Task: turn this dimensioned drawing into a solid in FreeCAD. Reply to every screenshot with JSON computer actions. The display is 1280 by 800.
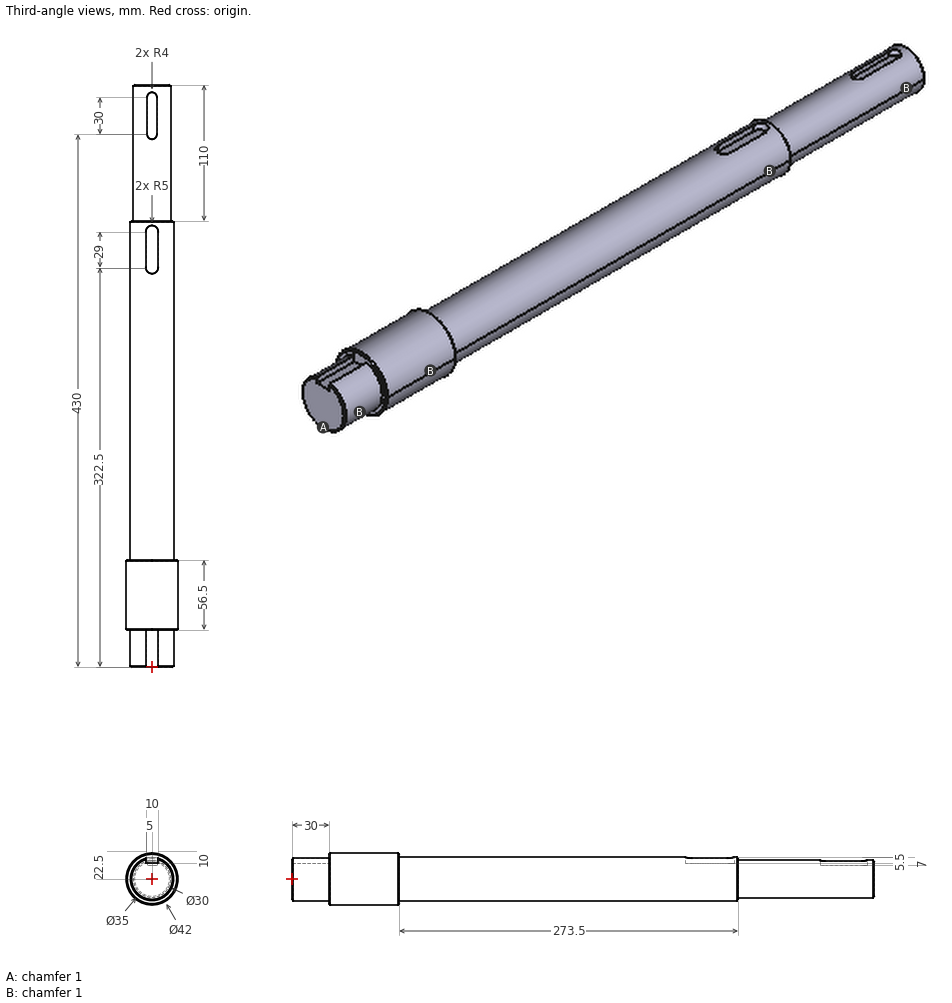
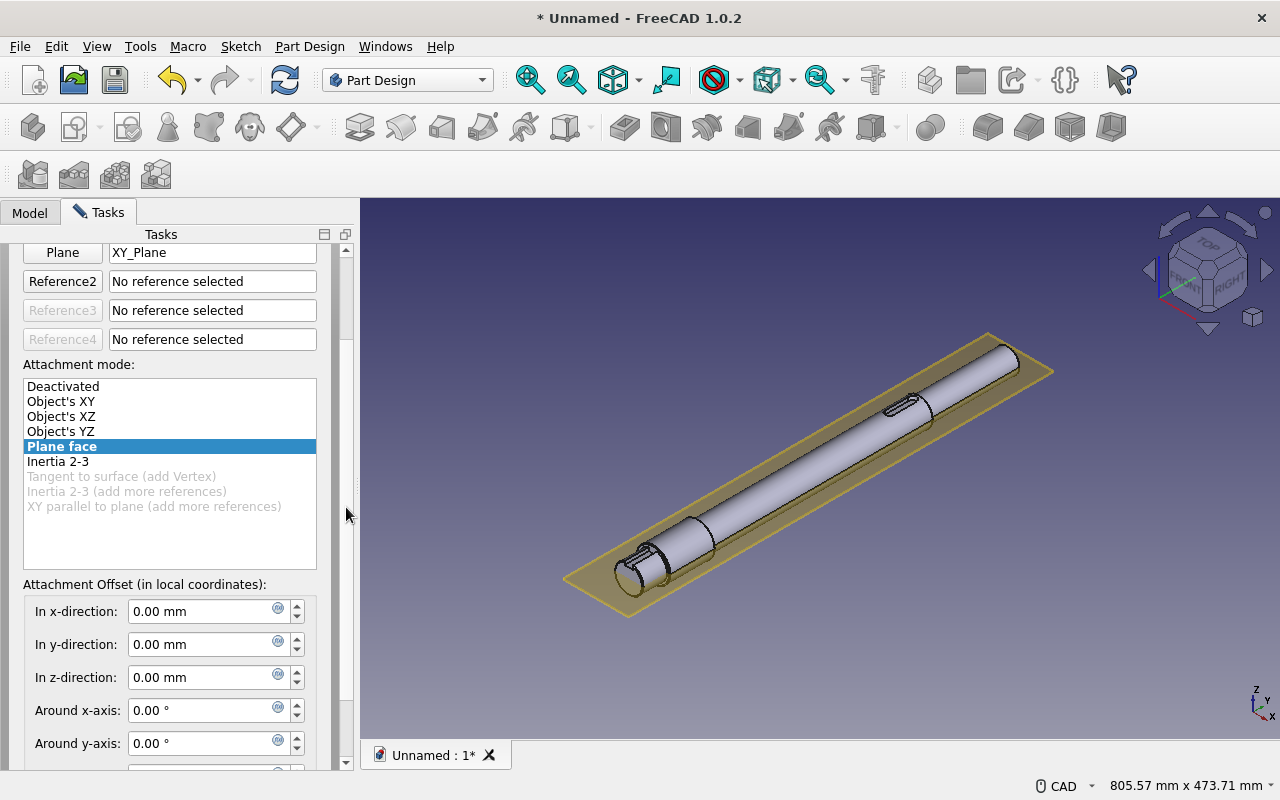
{"action": "triple_click", "coordinate": [210, 678]}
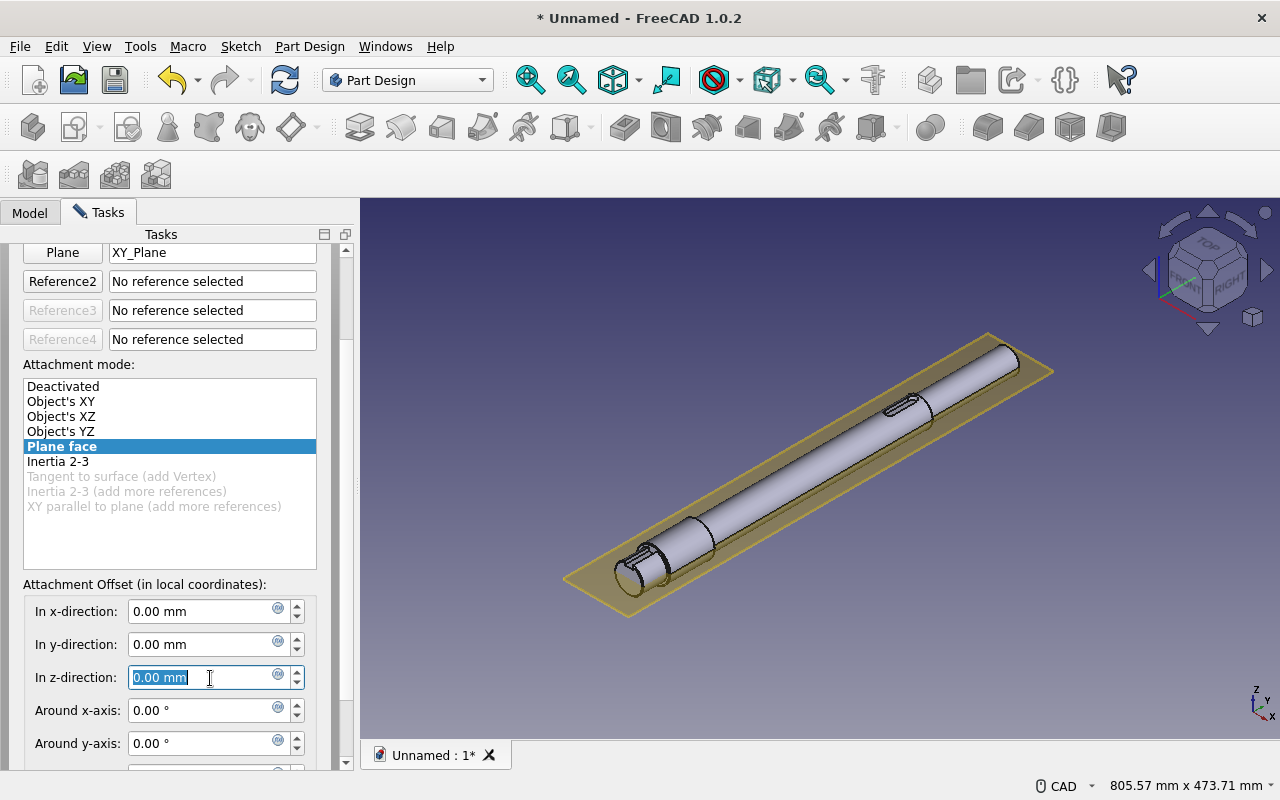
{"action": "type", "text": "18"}
{"action": "key", "text": "Tab"}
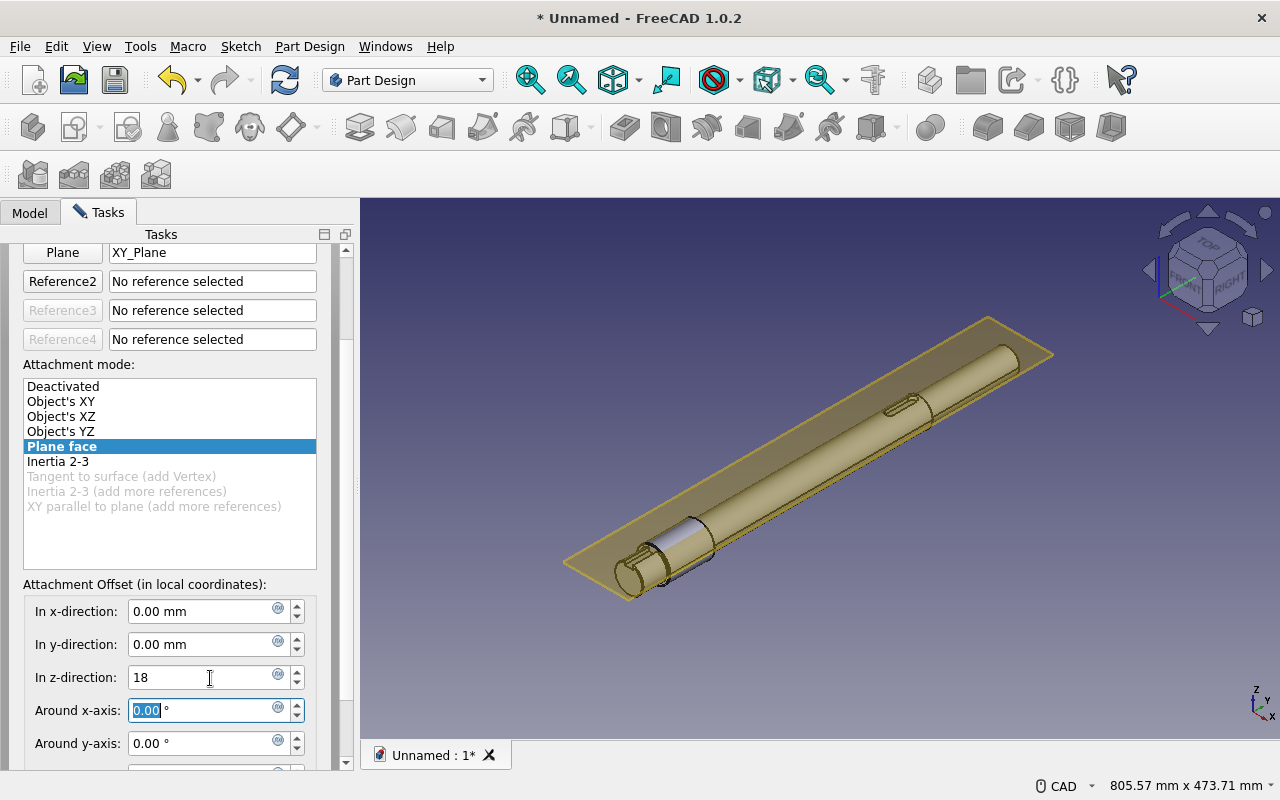
{"action": "scroll", "coordinate": [346, 507], "scroll_direction": "up", "scroll_amount": 3}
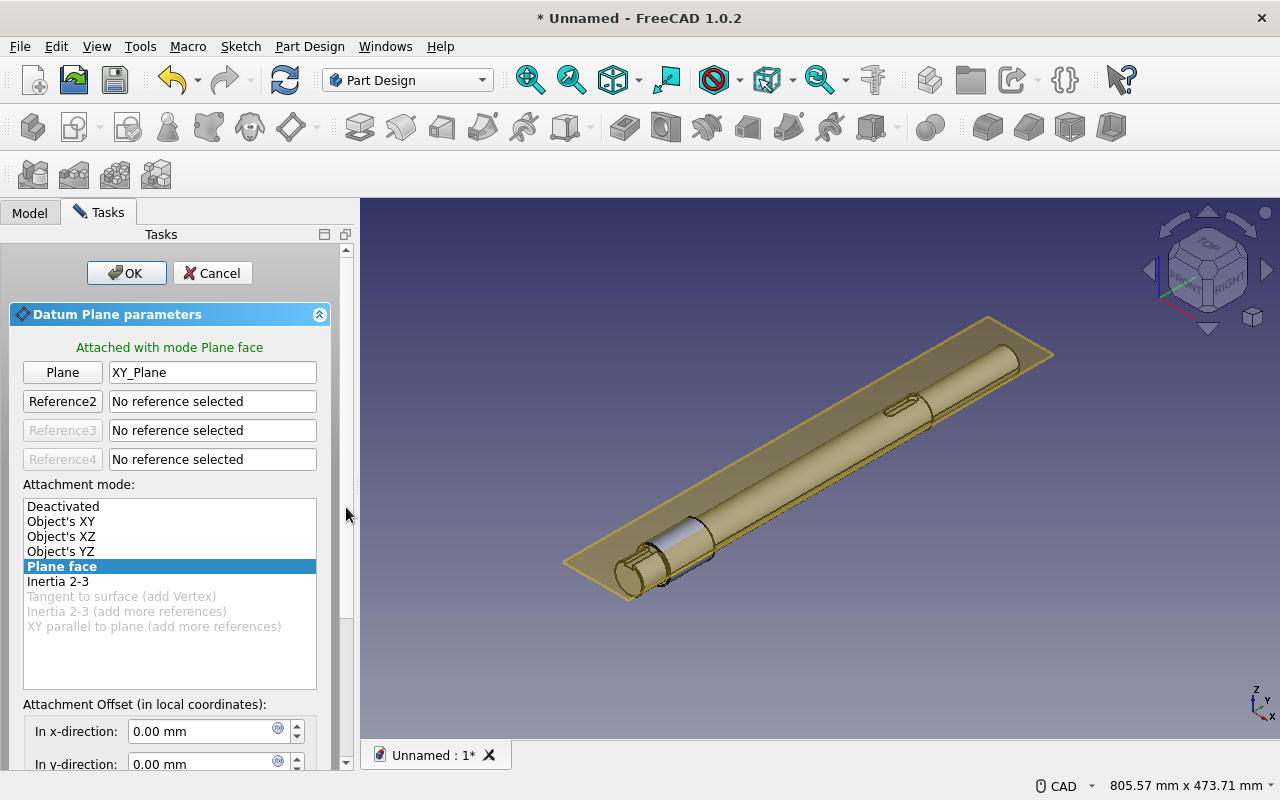
{"action": "left_click", "coordinate": [127, 273]}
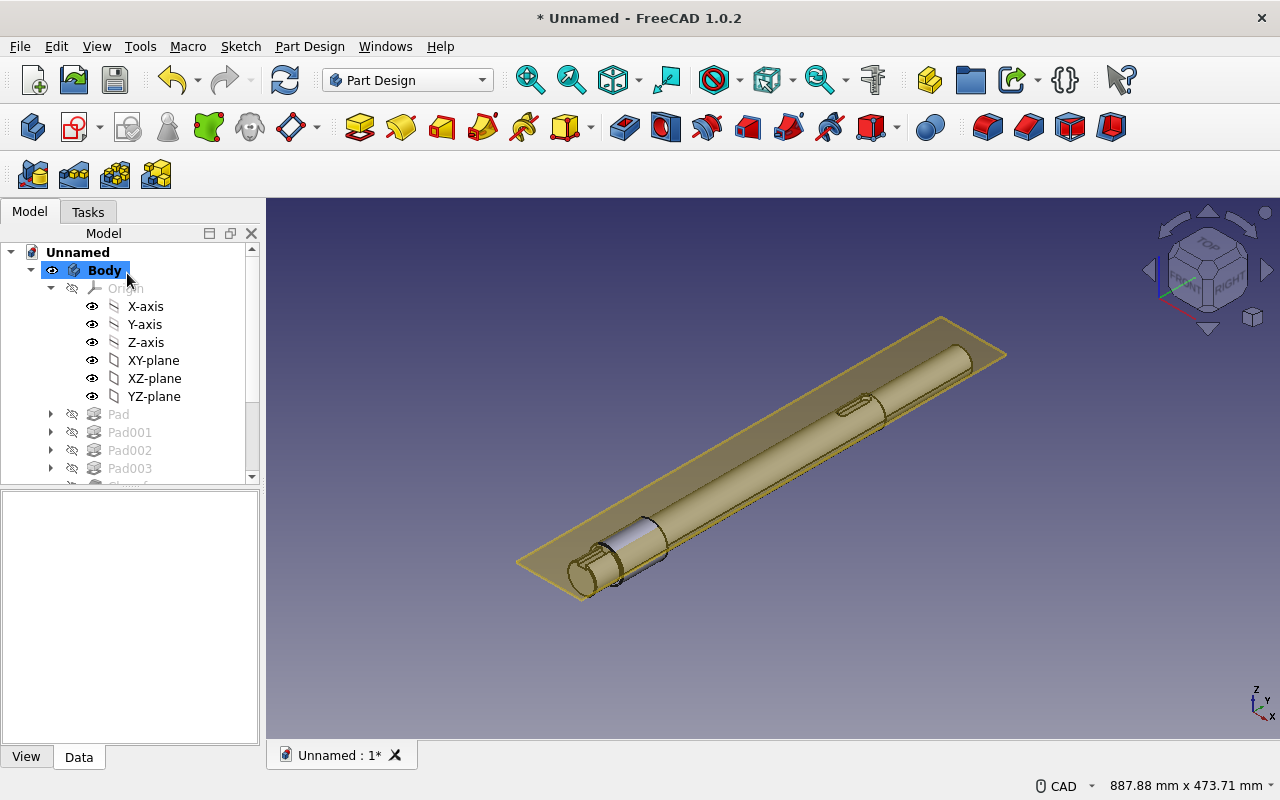
{"action": "scroll", "coordinate": [101, 356], "scroll_direction": "down", "scroll_amount": 3}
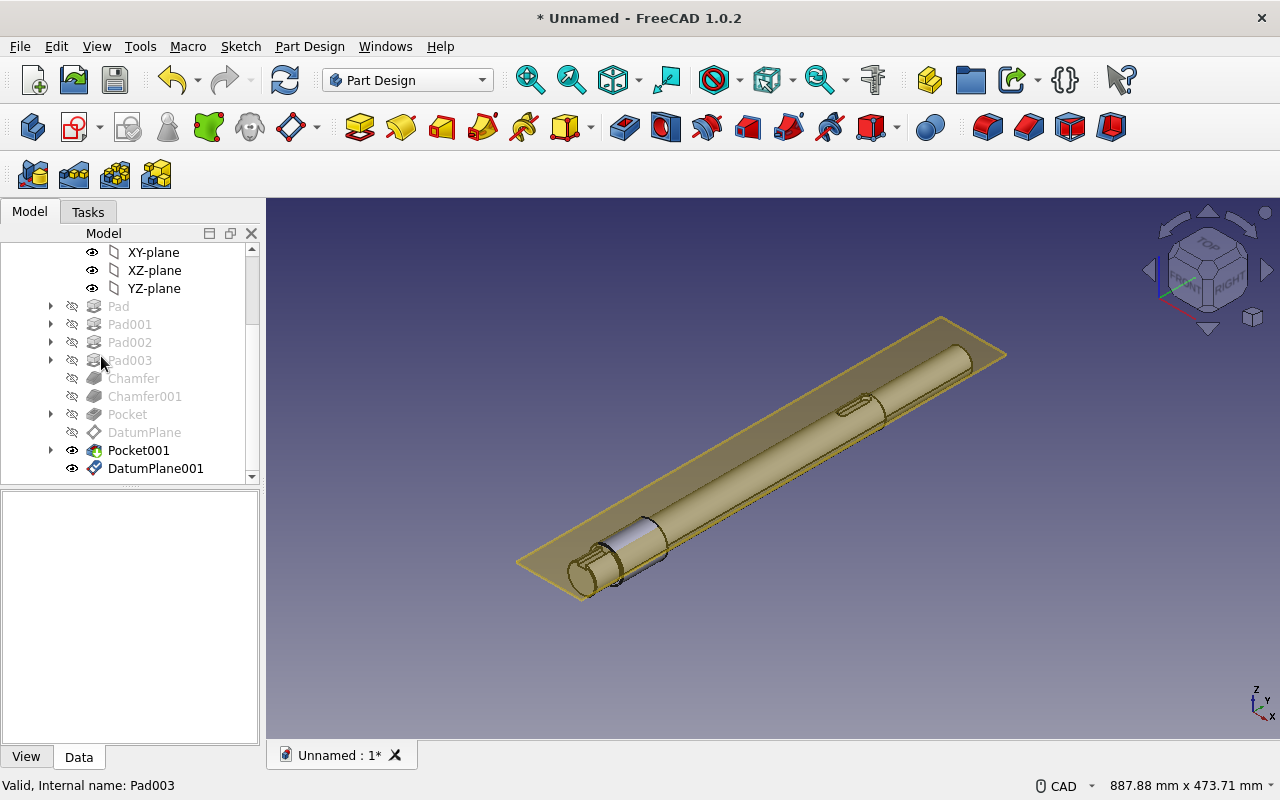
{"action": "left_click", "coordinate": [117, 468]}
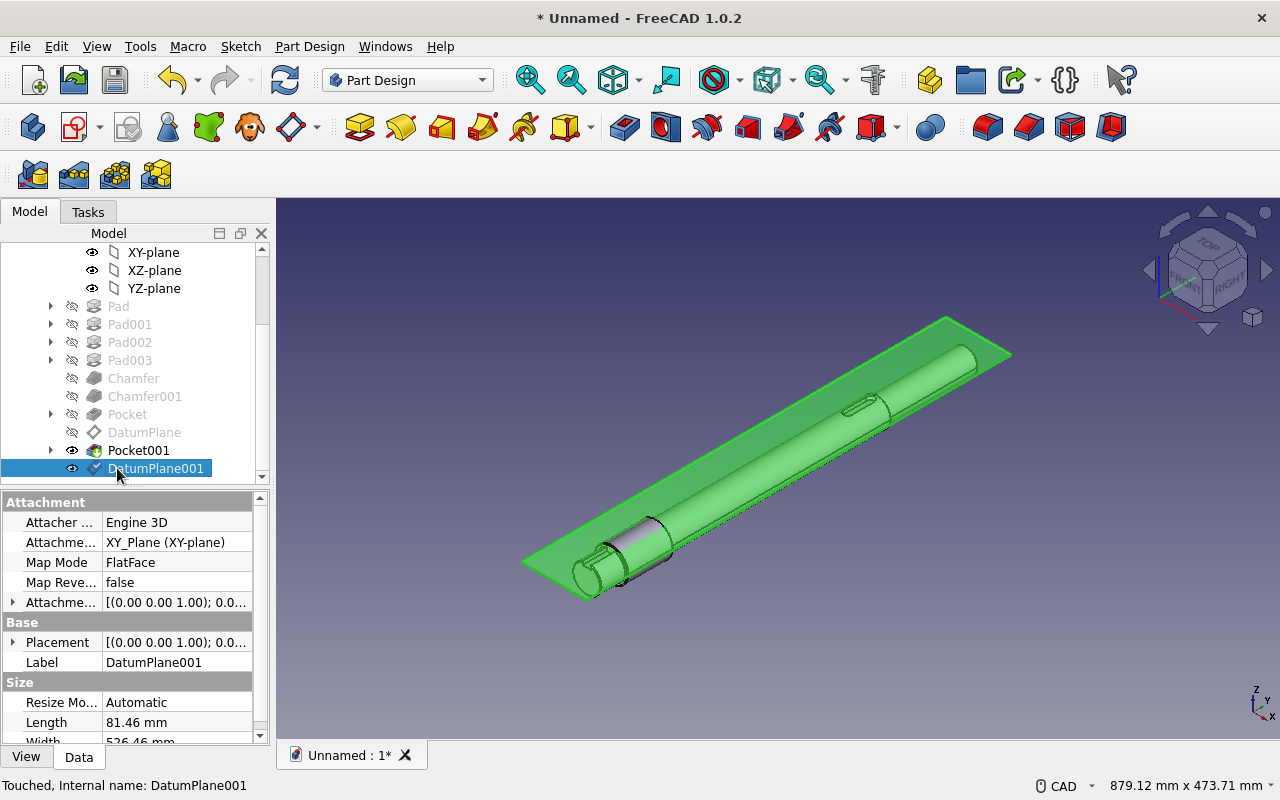
{"action": "left_click", "coordinate": [74, 128]}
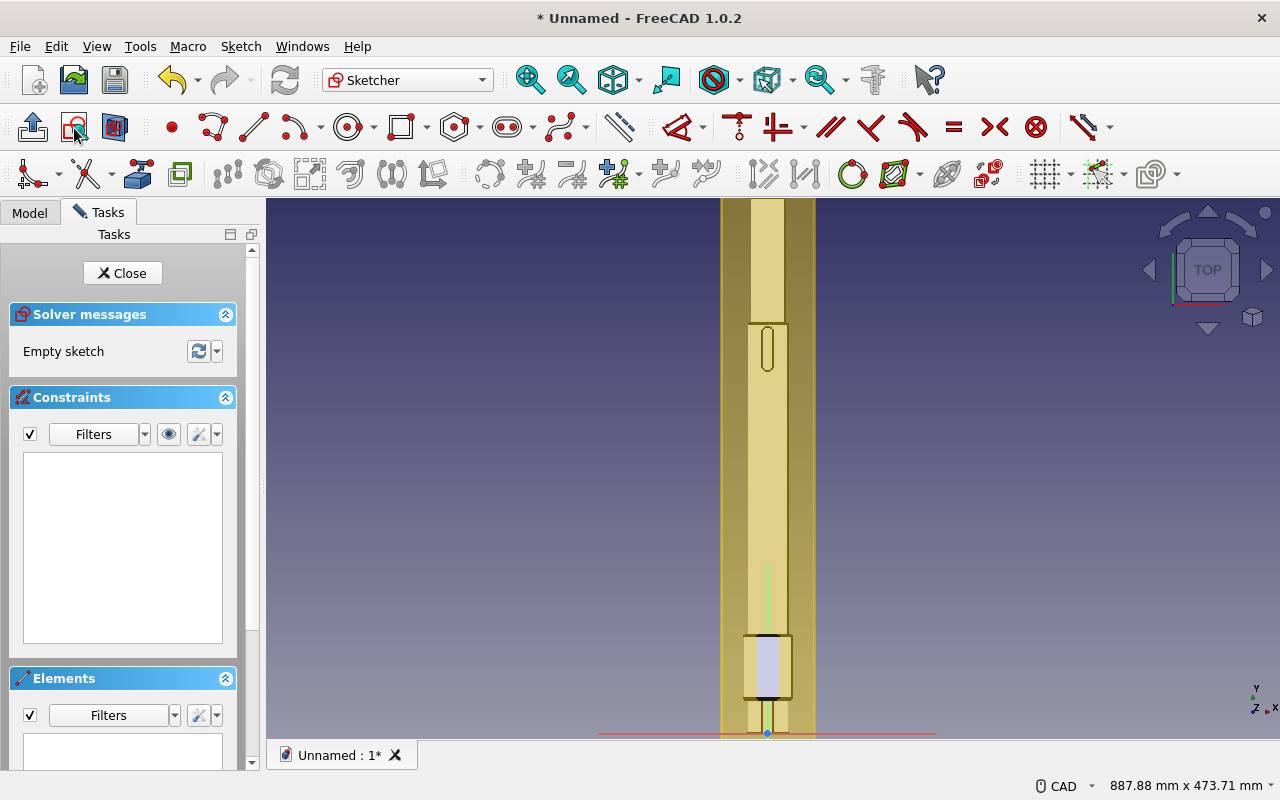
{"action": "key", "text": "q s"}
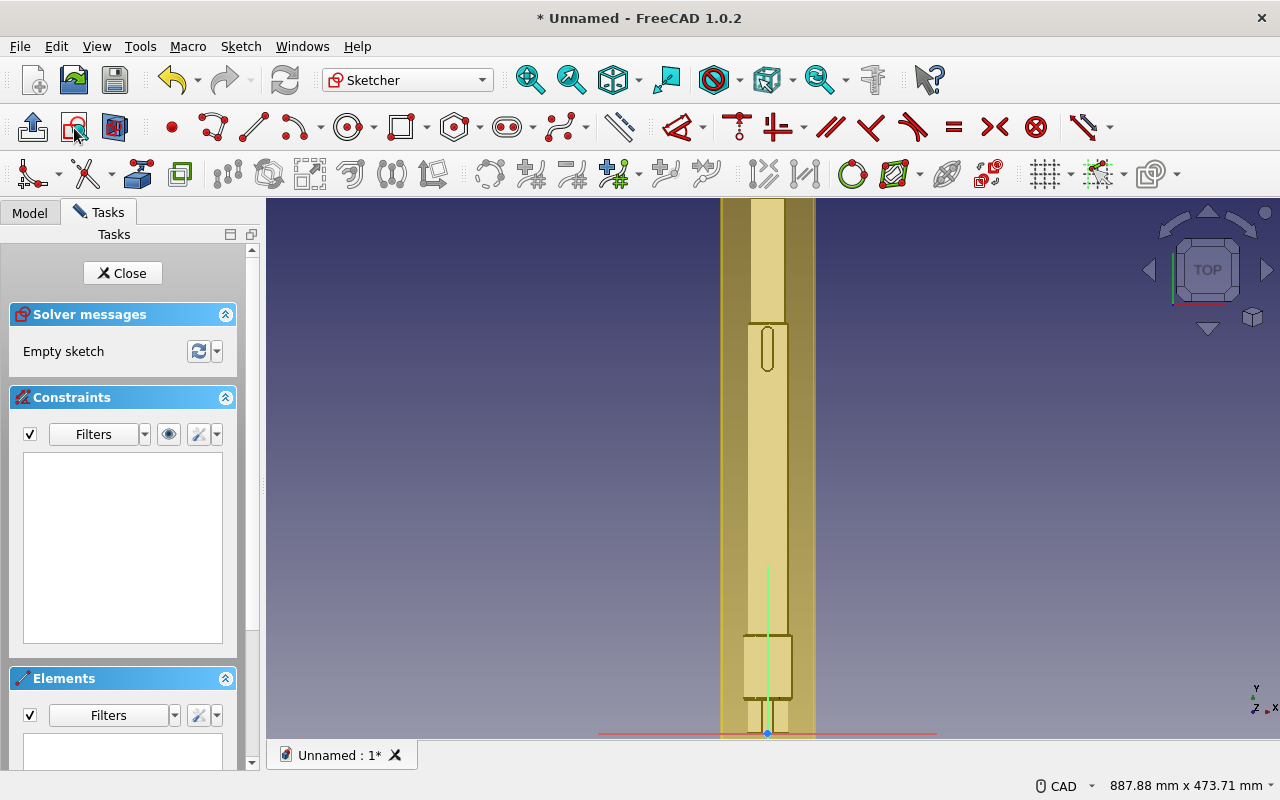
{"action": "scroll", "coordinate": [704, 468], "scroll_direction": "down", "scroll_amount": 5}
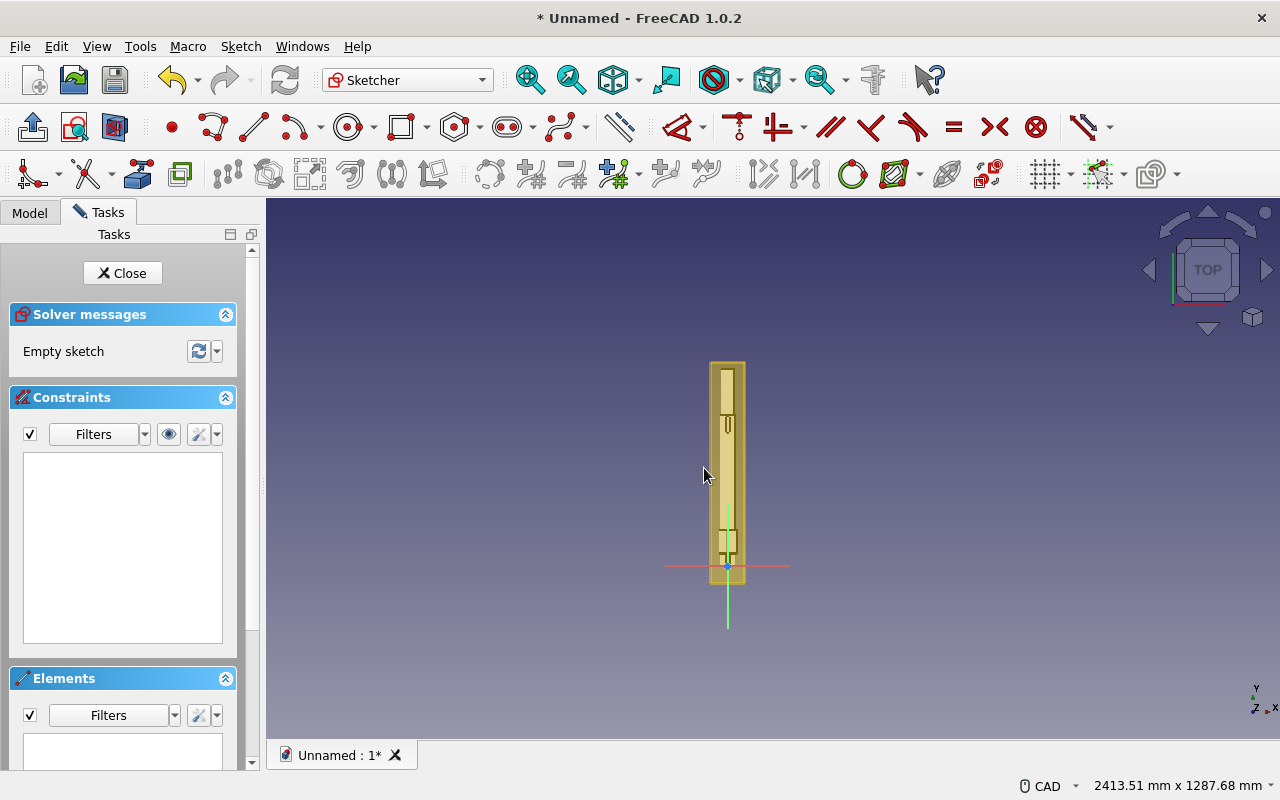
{"action": "scroll", "coordinate": [729, 374], "scroll_direction": "up", "scroll_amount": 15}